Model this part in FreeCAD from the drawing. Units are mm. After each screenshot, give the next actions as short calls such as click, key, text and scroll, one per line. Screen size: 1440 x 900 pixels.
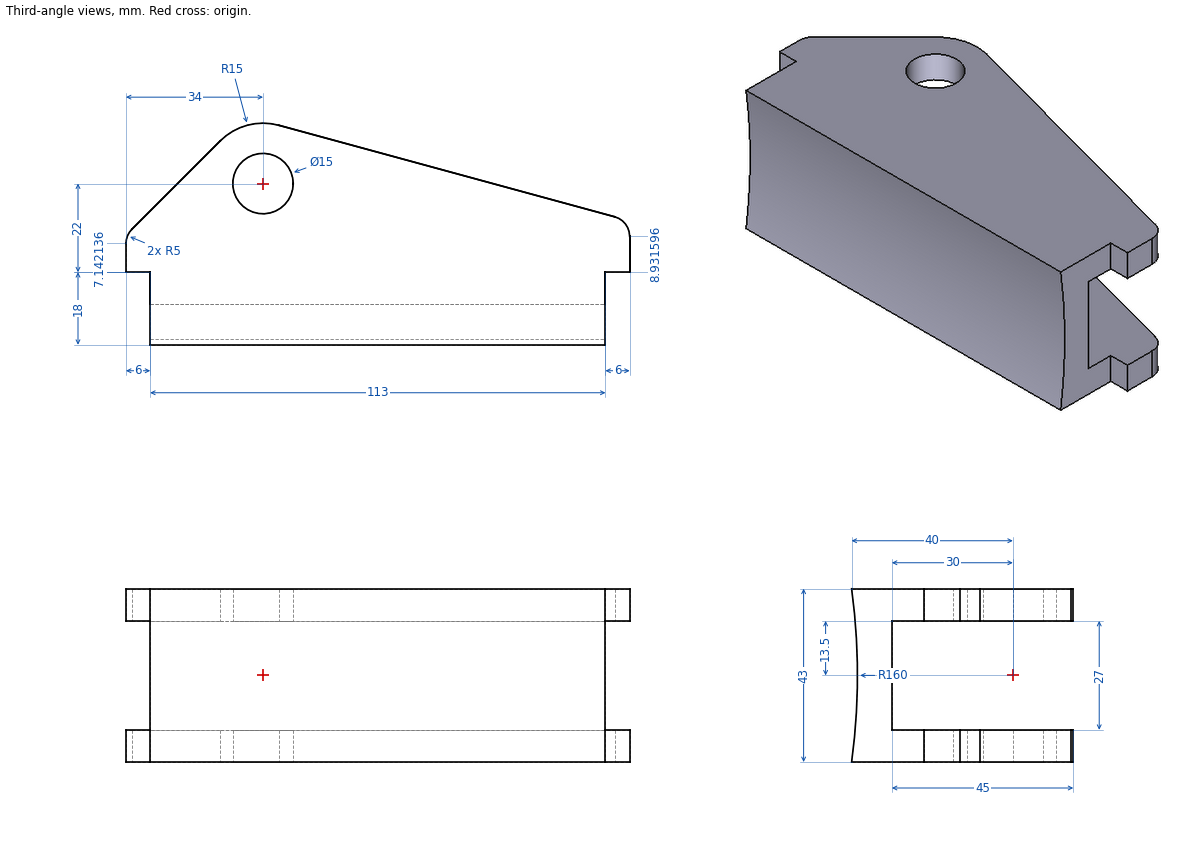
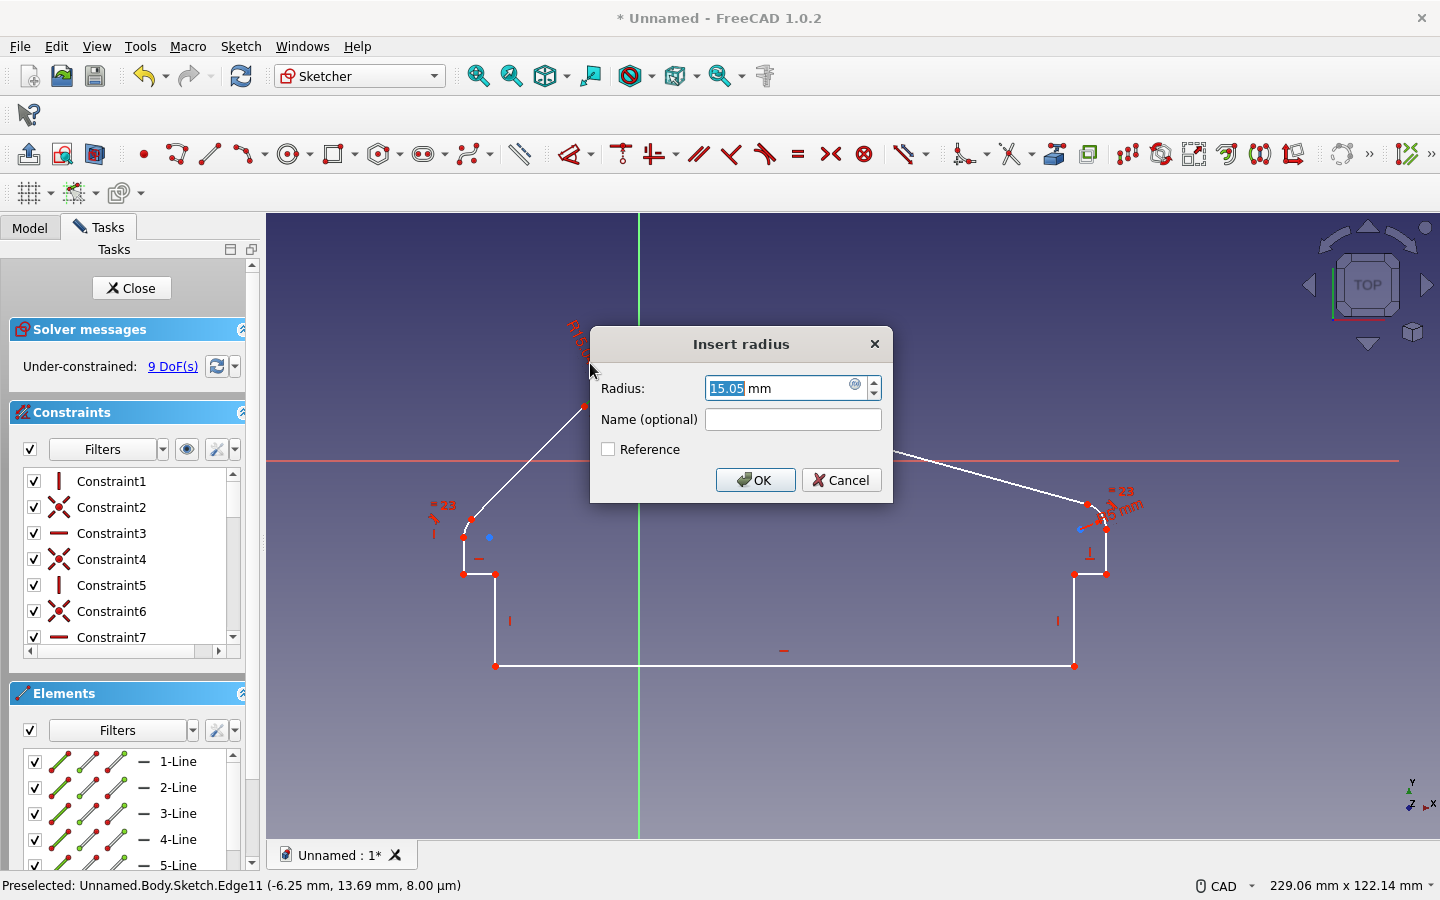
text(15)
key(Return)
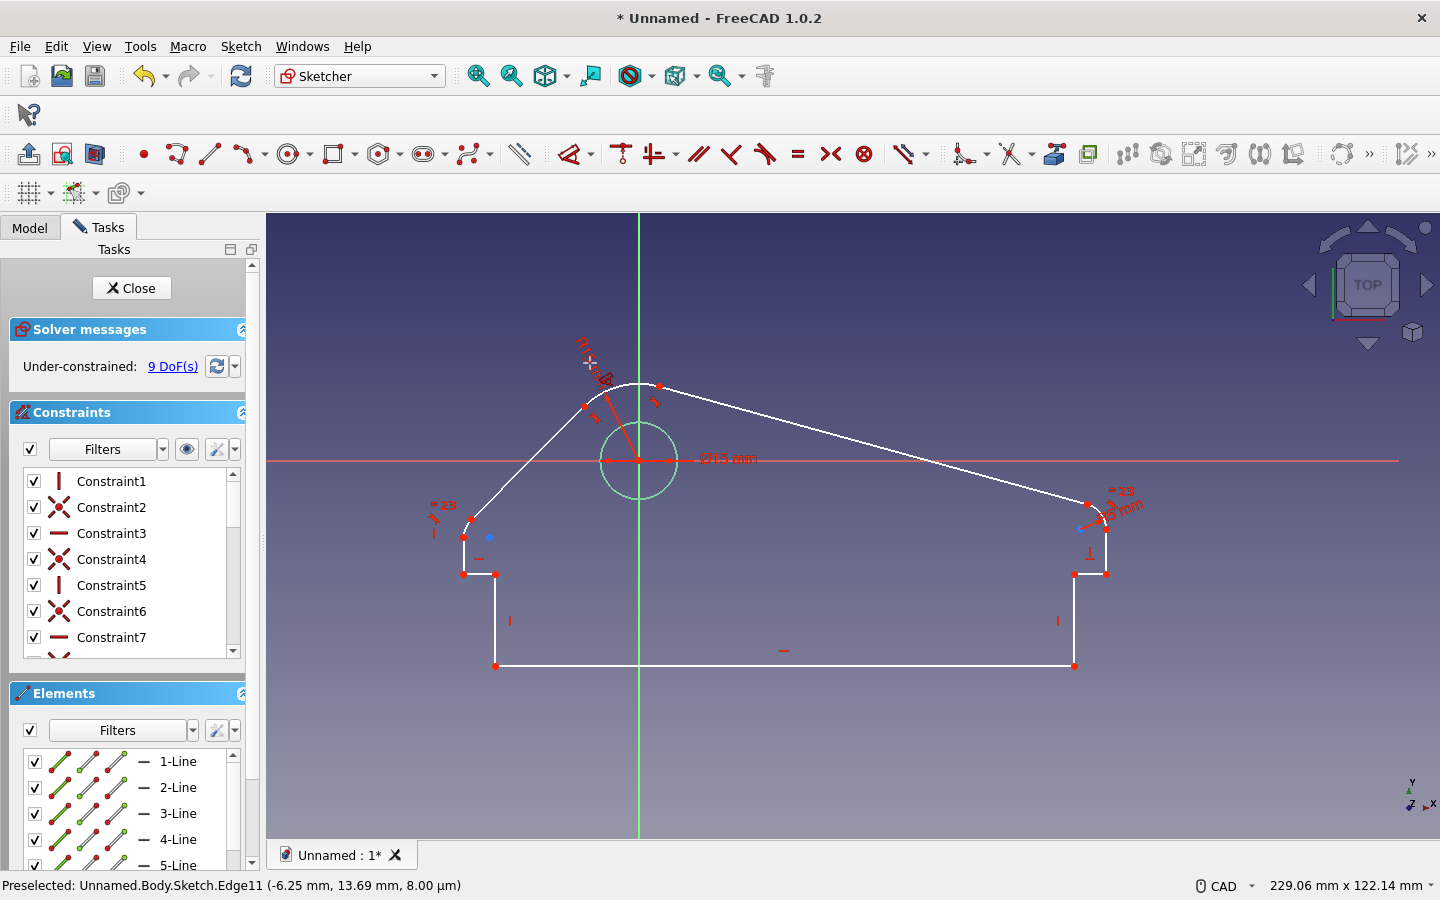
scroll(473, 574, up, 2)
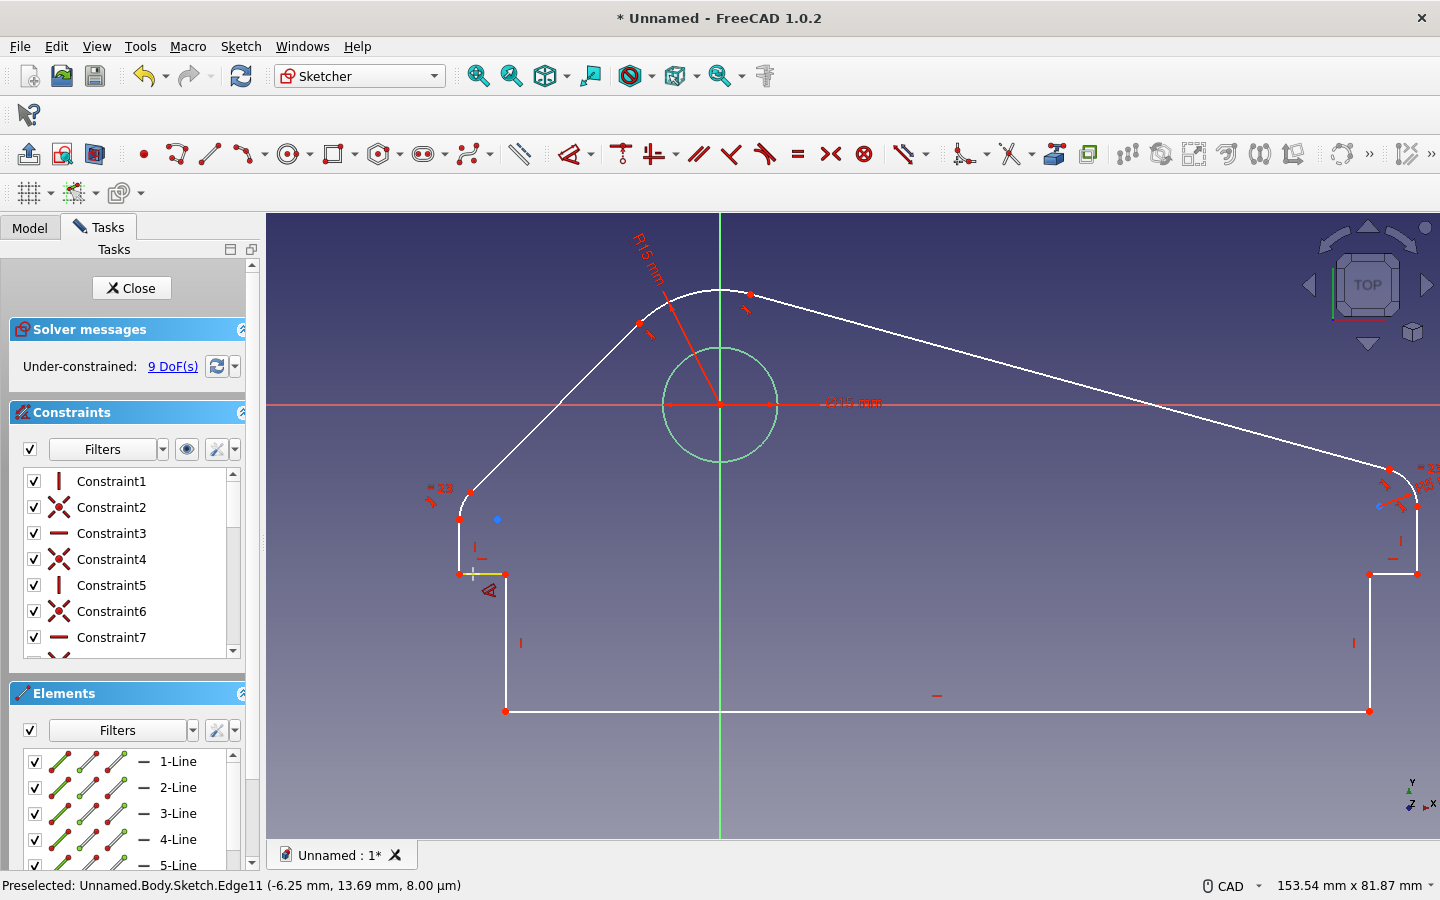
click(473, 574)
click(483, 608)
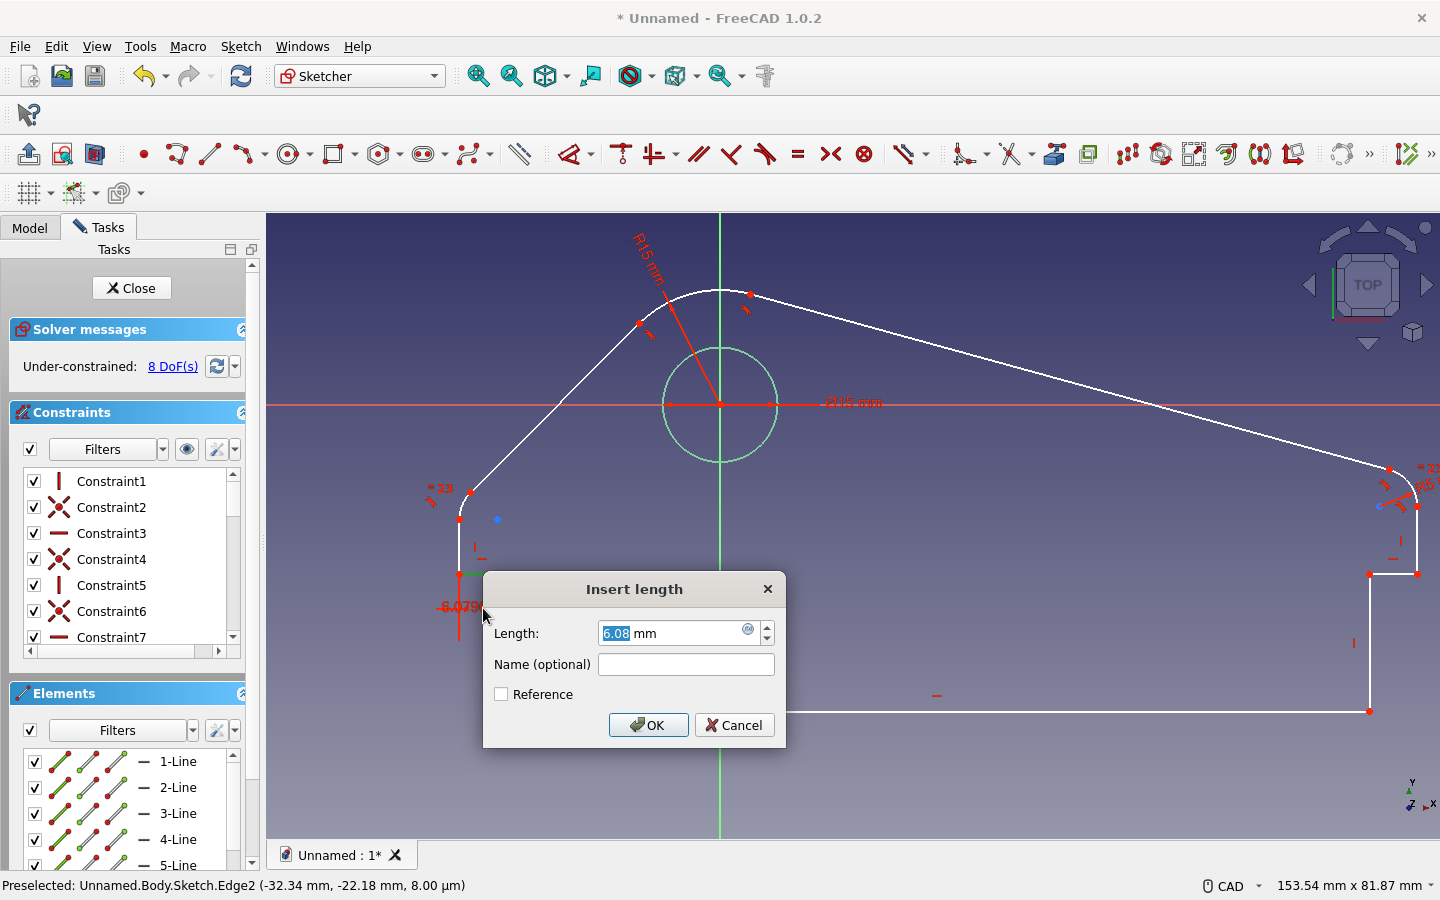
text(6)
key(Return)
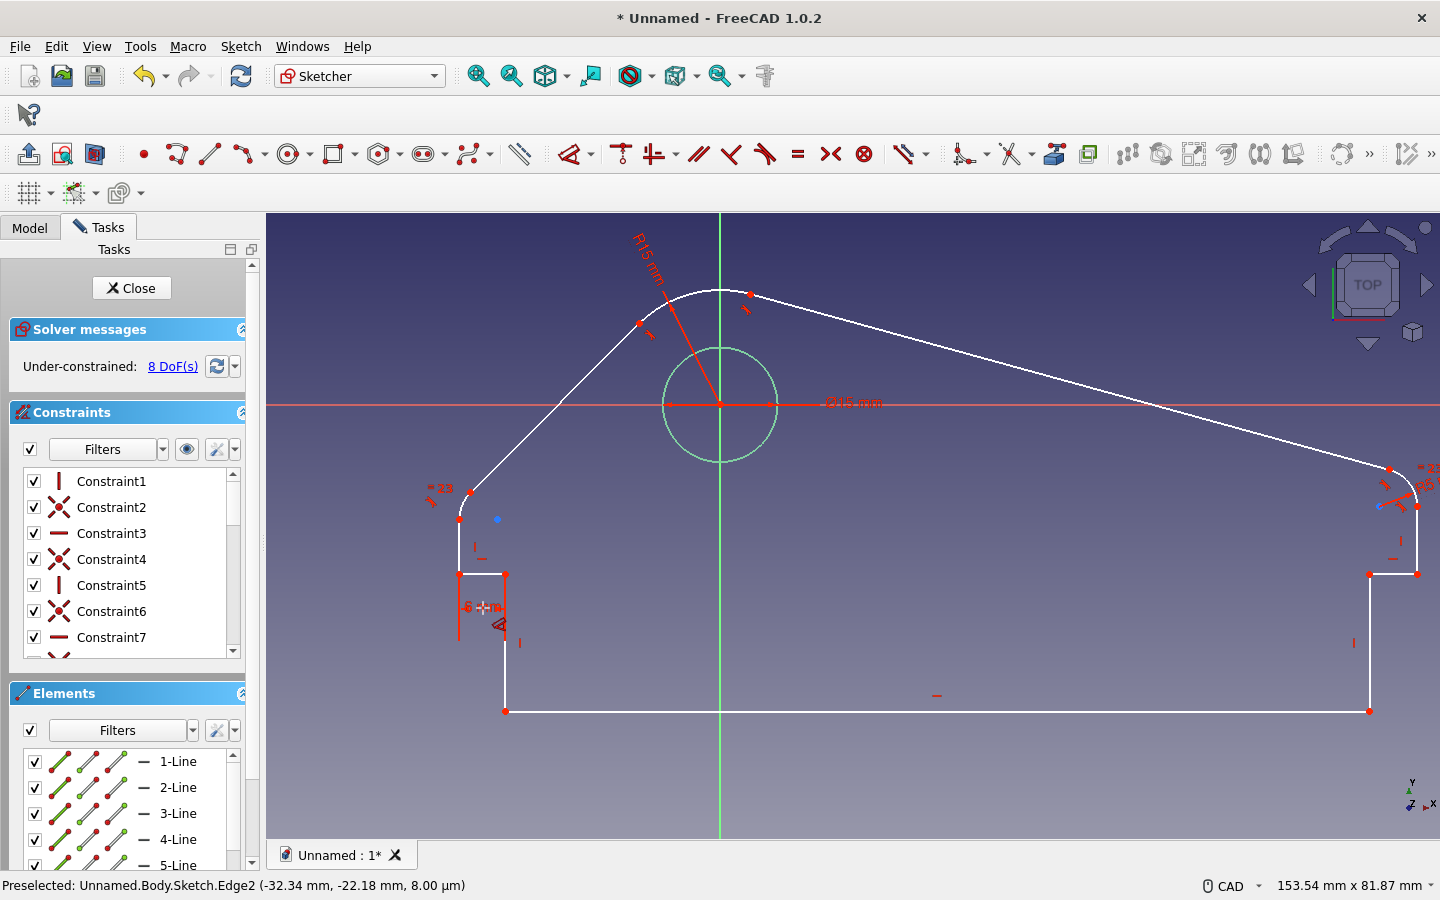
scroll(472, 574, down, 2)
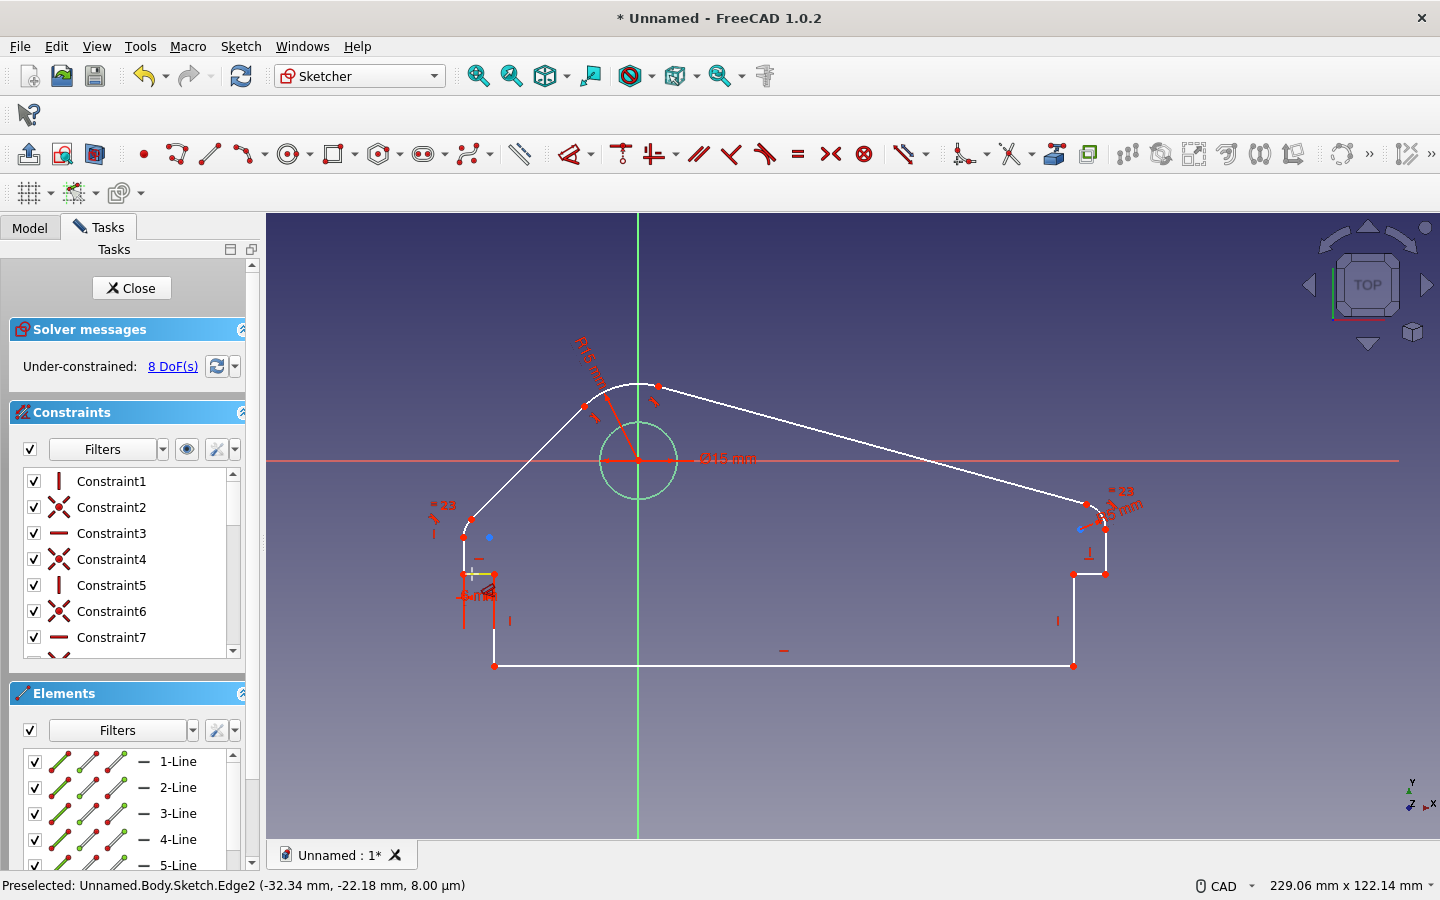
scroll(1083, 574, up, 2)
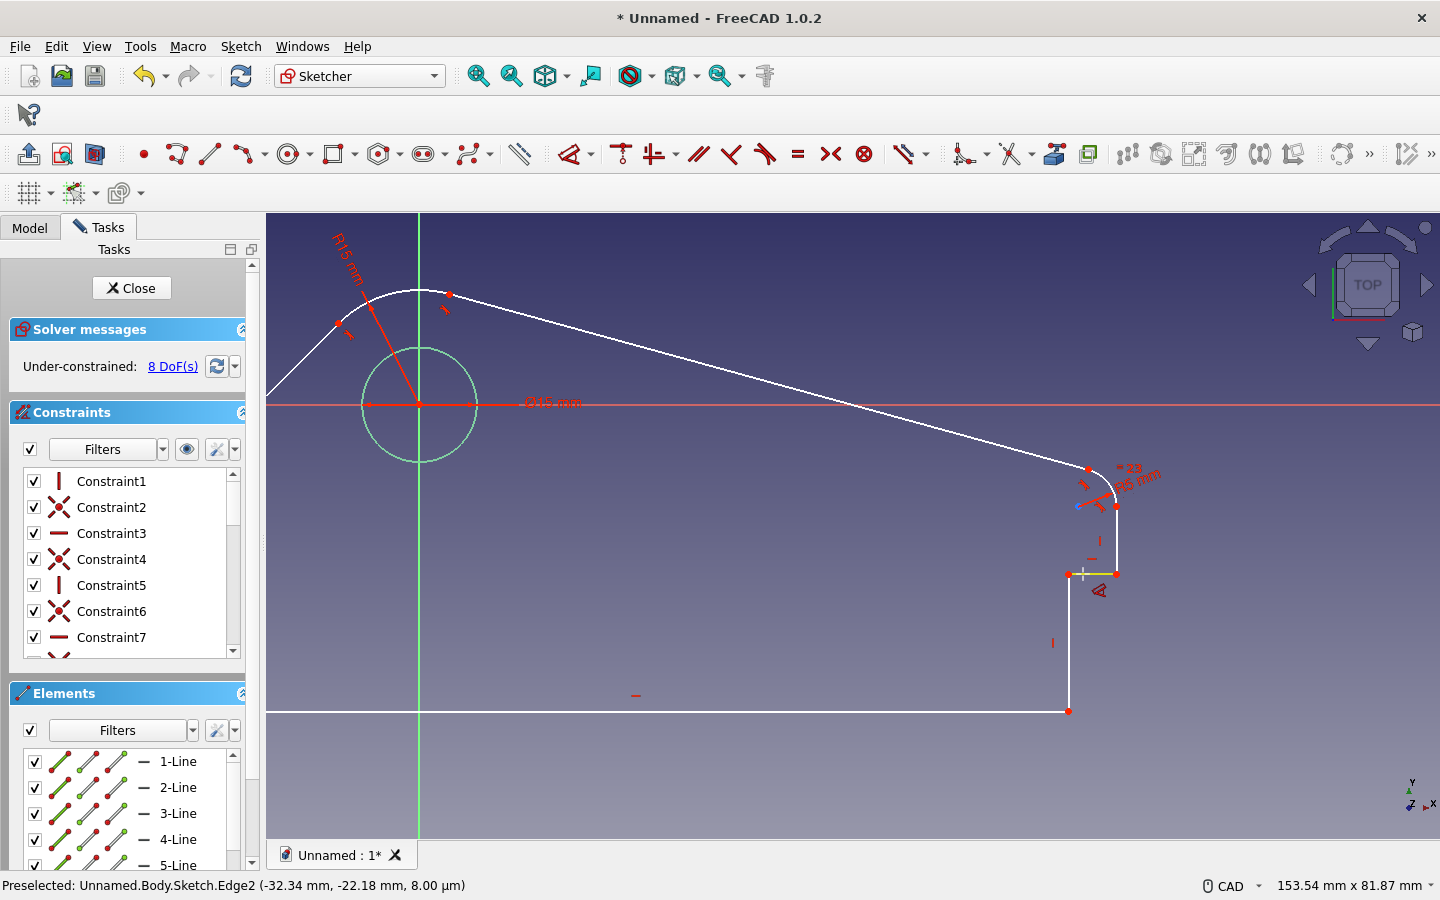
click(1083, 574)
click(1093, 608)